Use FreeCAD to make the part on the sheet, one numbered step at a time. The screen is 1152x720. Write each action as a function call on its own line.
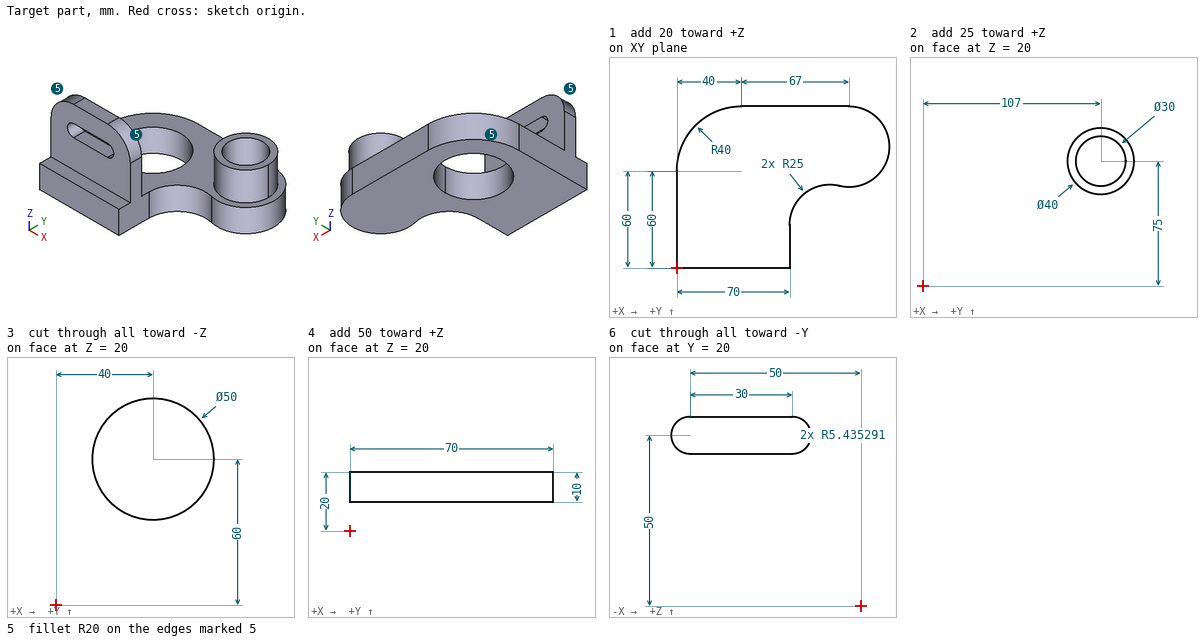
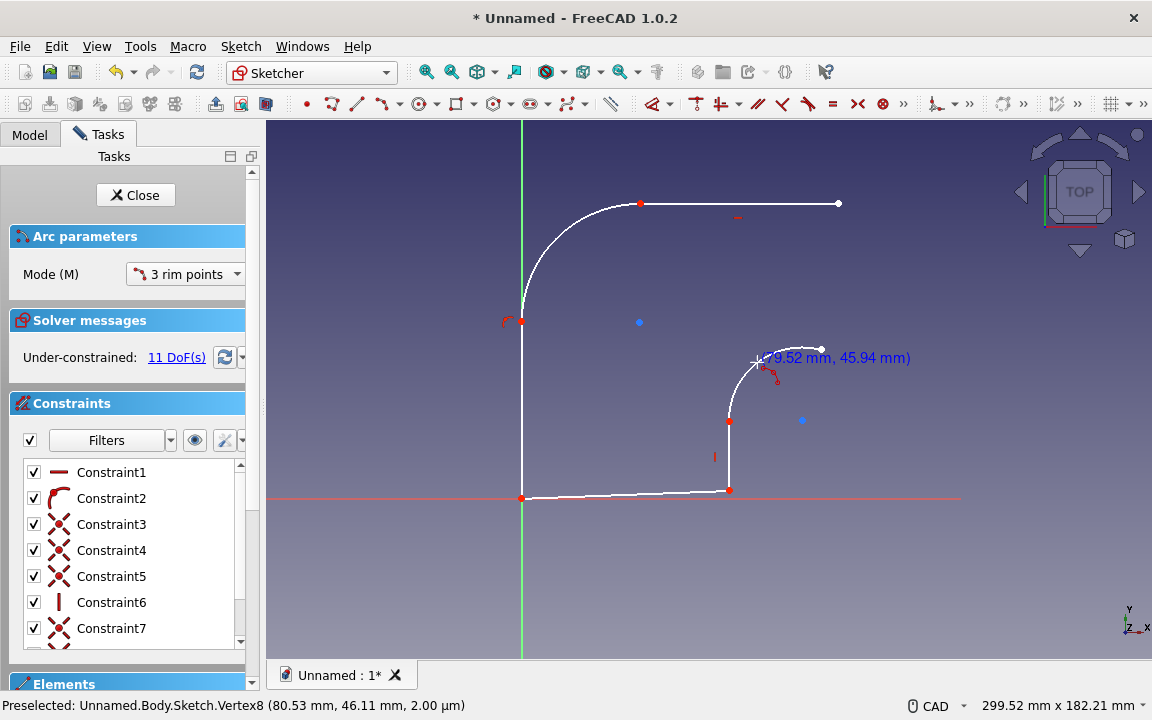
click(821, 350)
click(838, 204)
click(912, 286)
key(Escape)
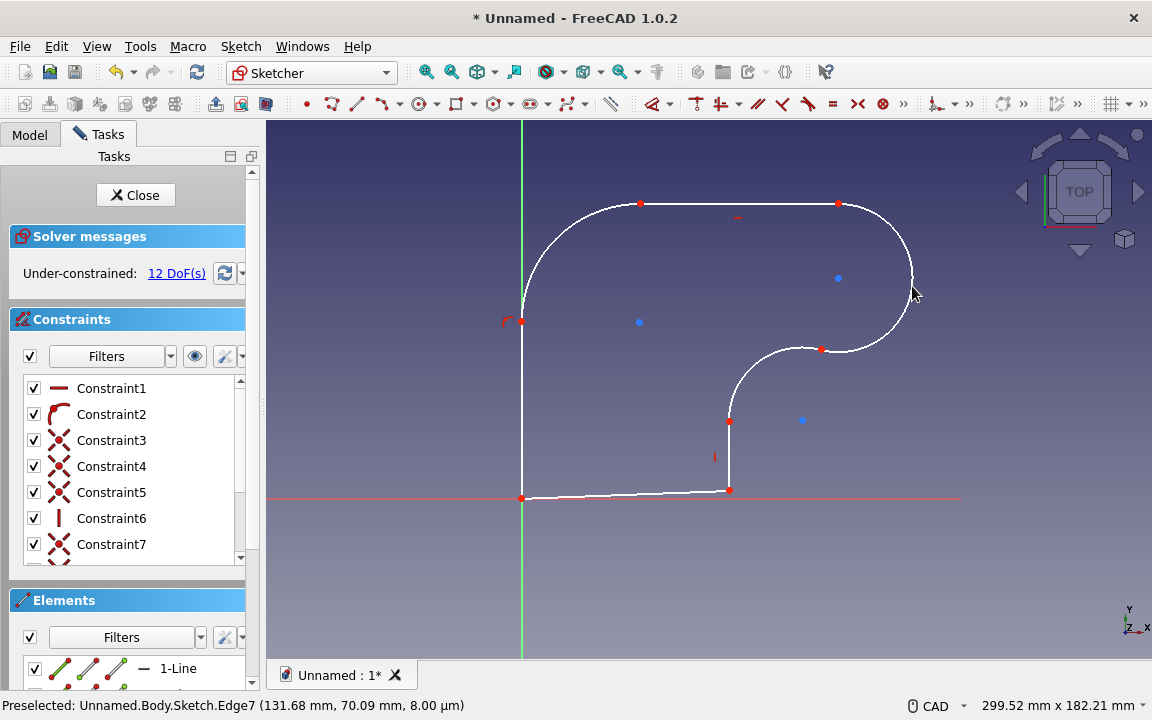
click(779, 204)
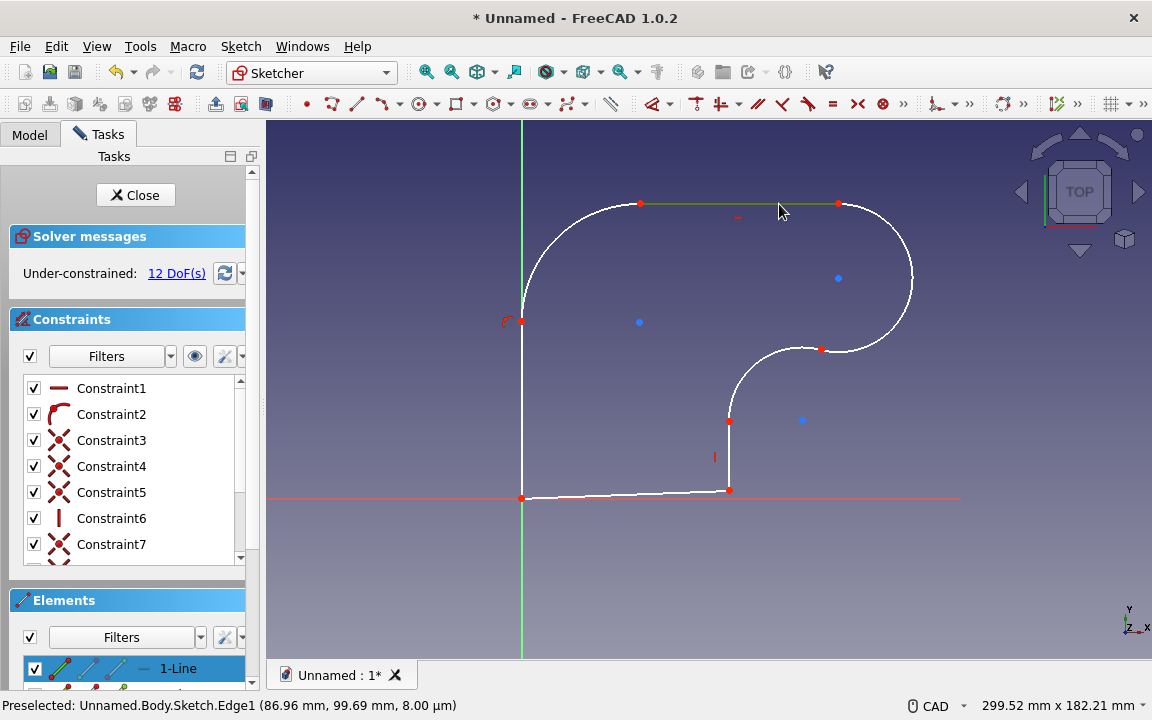
click(890, 331)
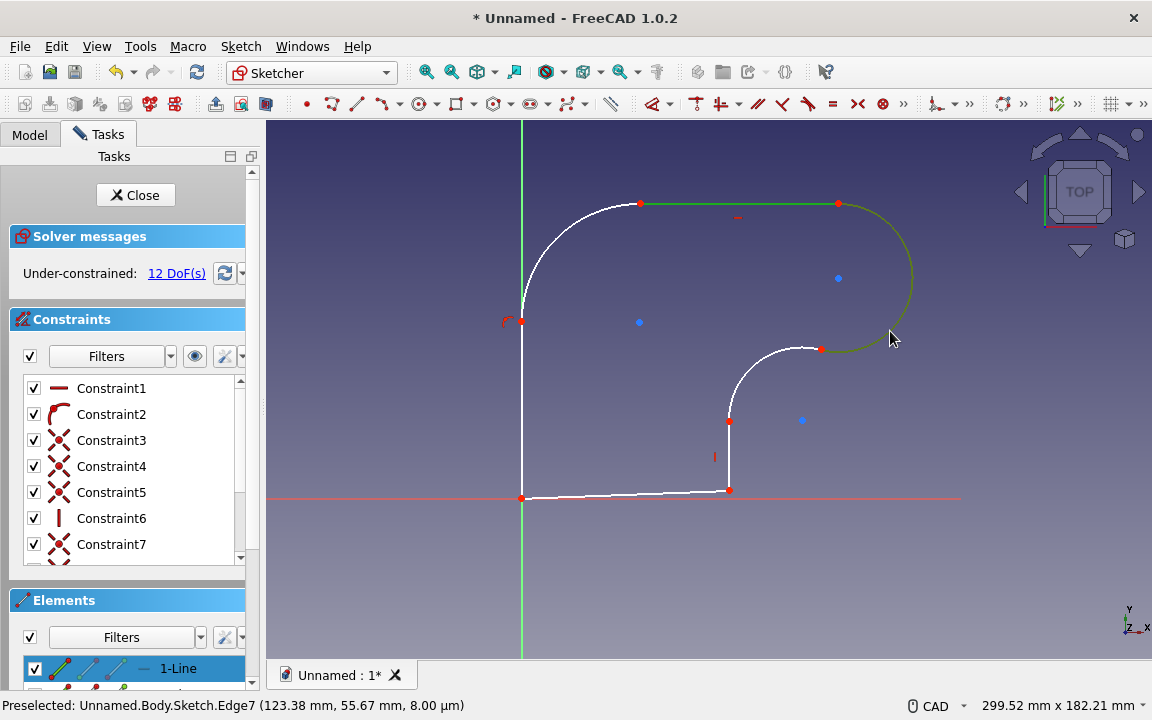
click(808, 104)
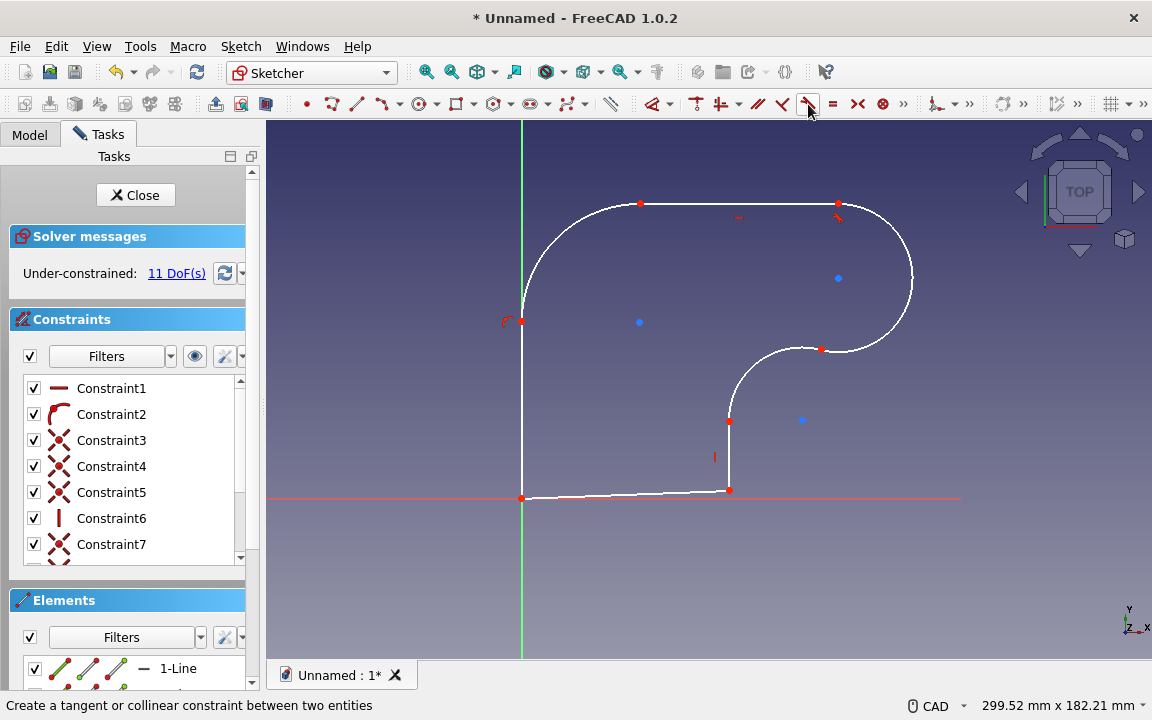
click(729, 470)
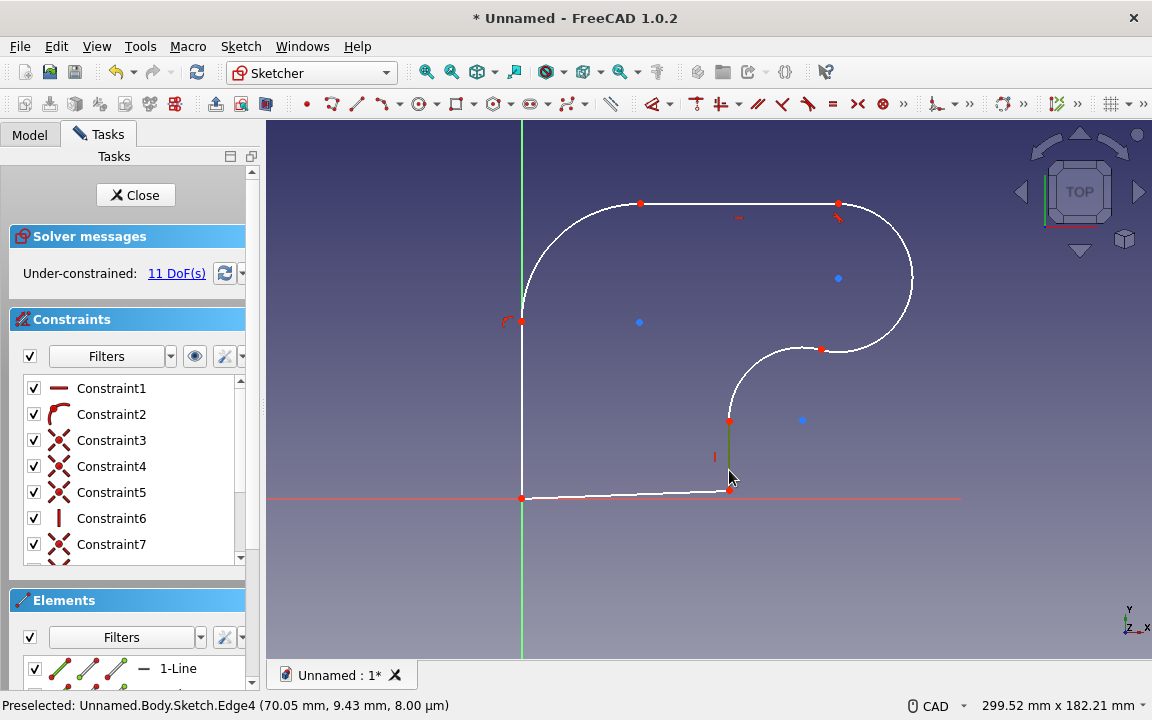
click(781, 351)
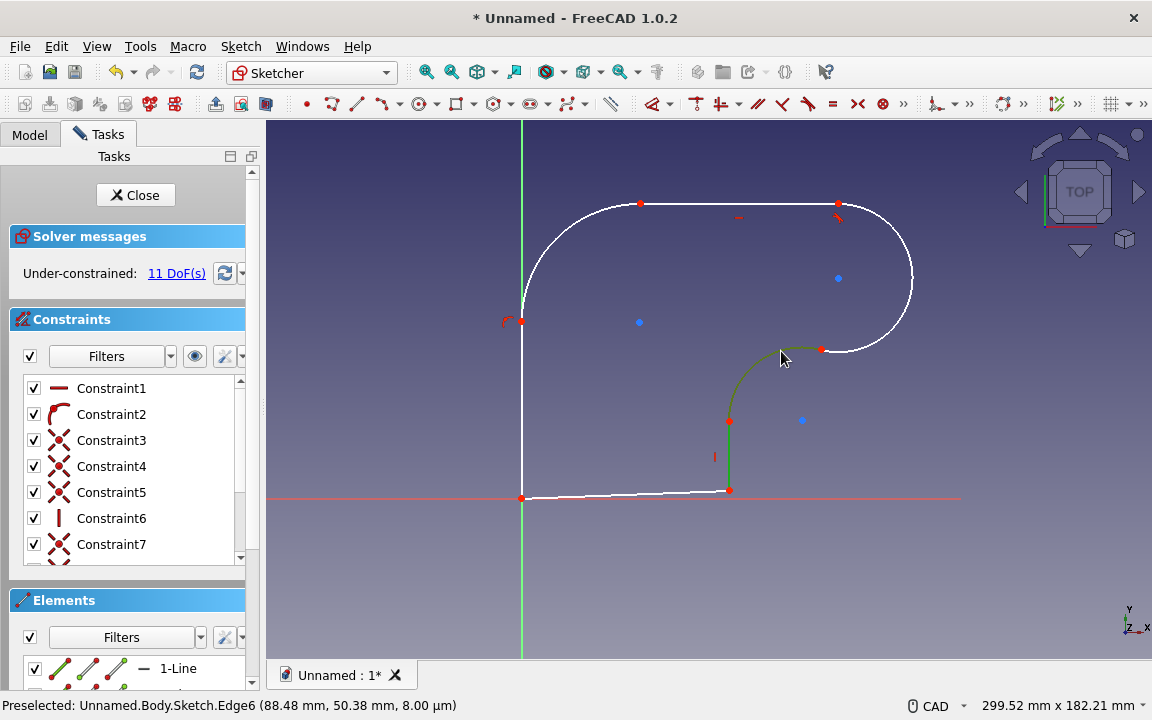
click(808, 104)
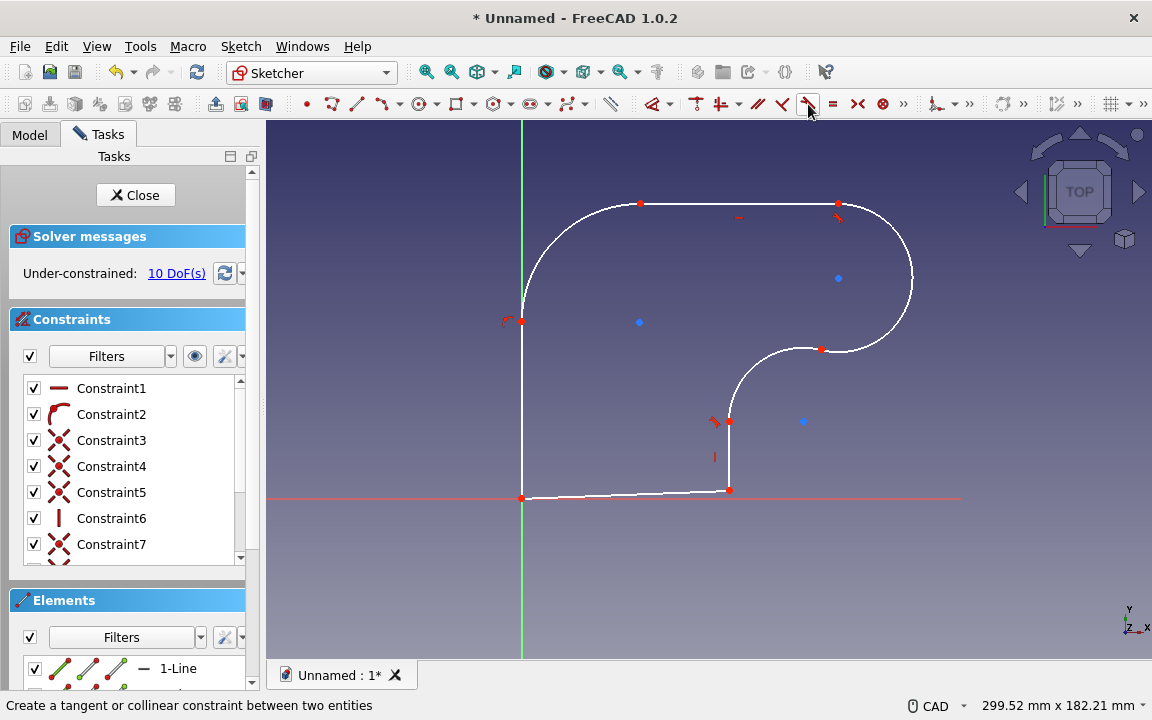
click(781, 351)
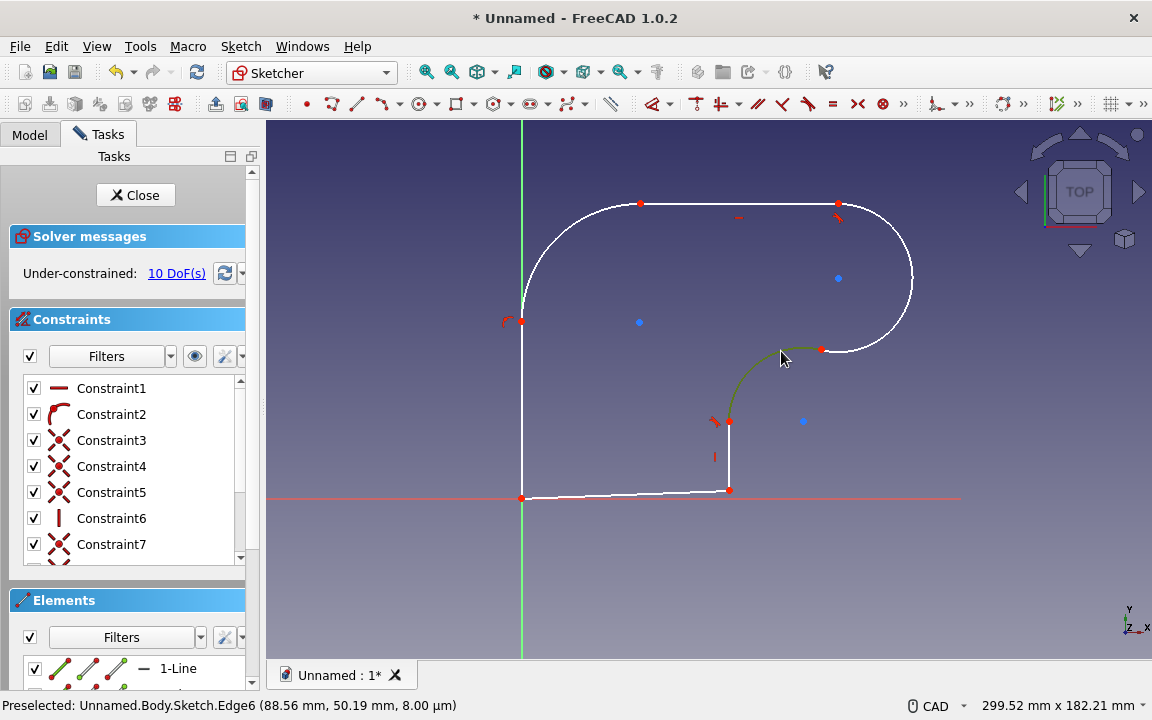
click(890, 331)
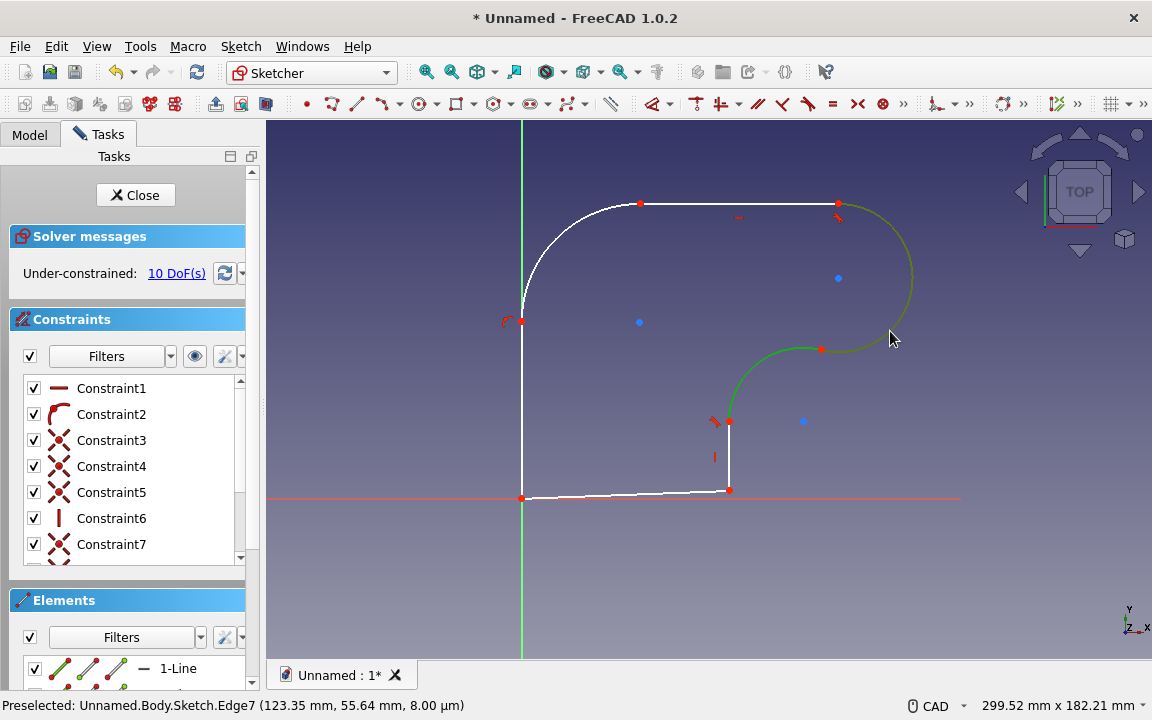
click(808, 104)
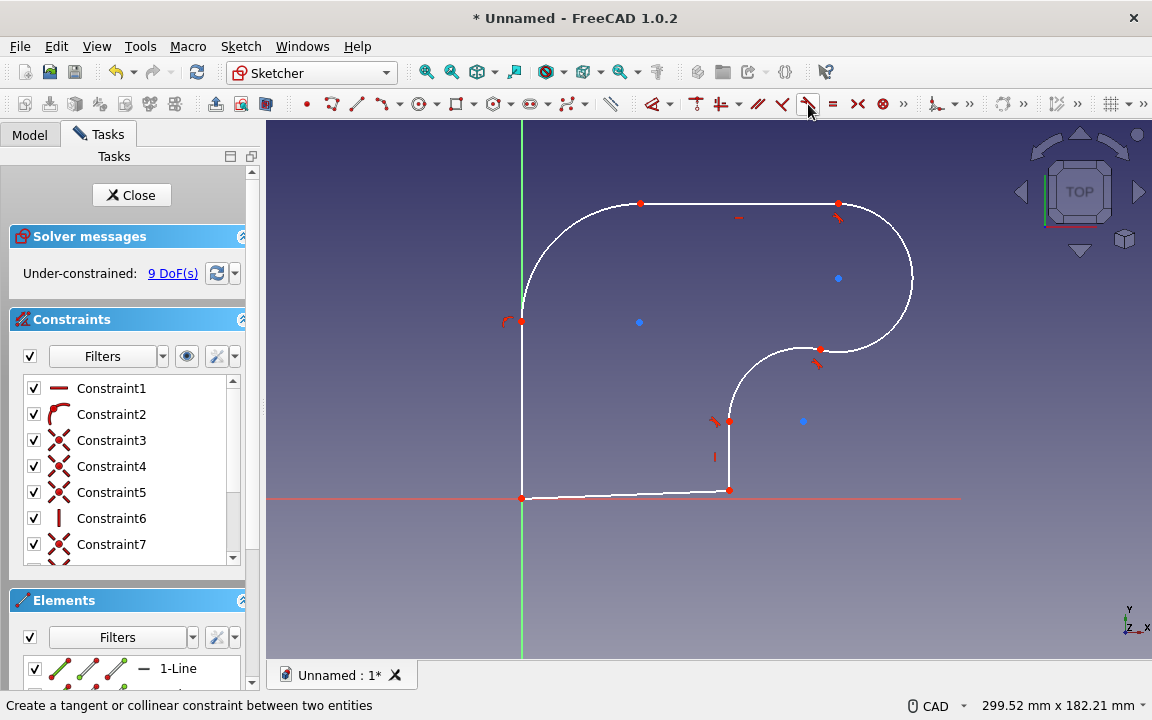
click(584, 497)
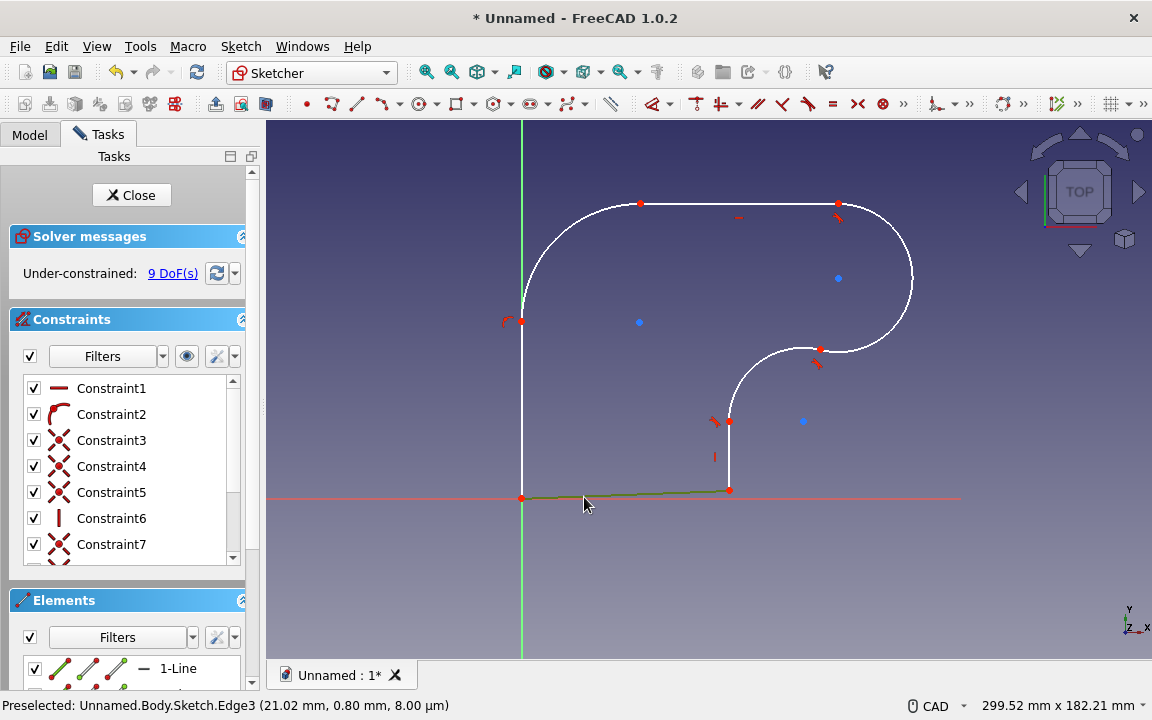
key(h)